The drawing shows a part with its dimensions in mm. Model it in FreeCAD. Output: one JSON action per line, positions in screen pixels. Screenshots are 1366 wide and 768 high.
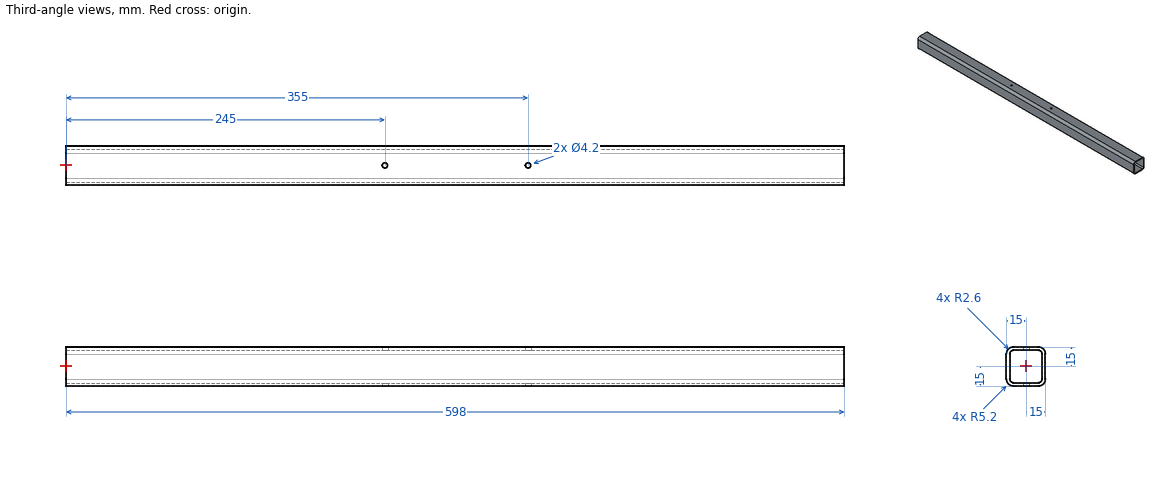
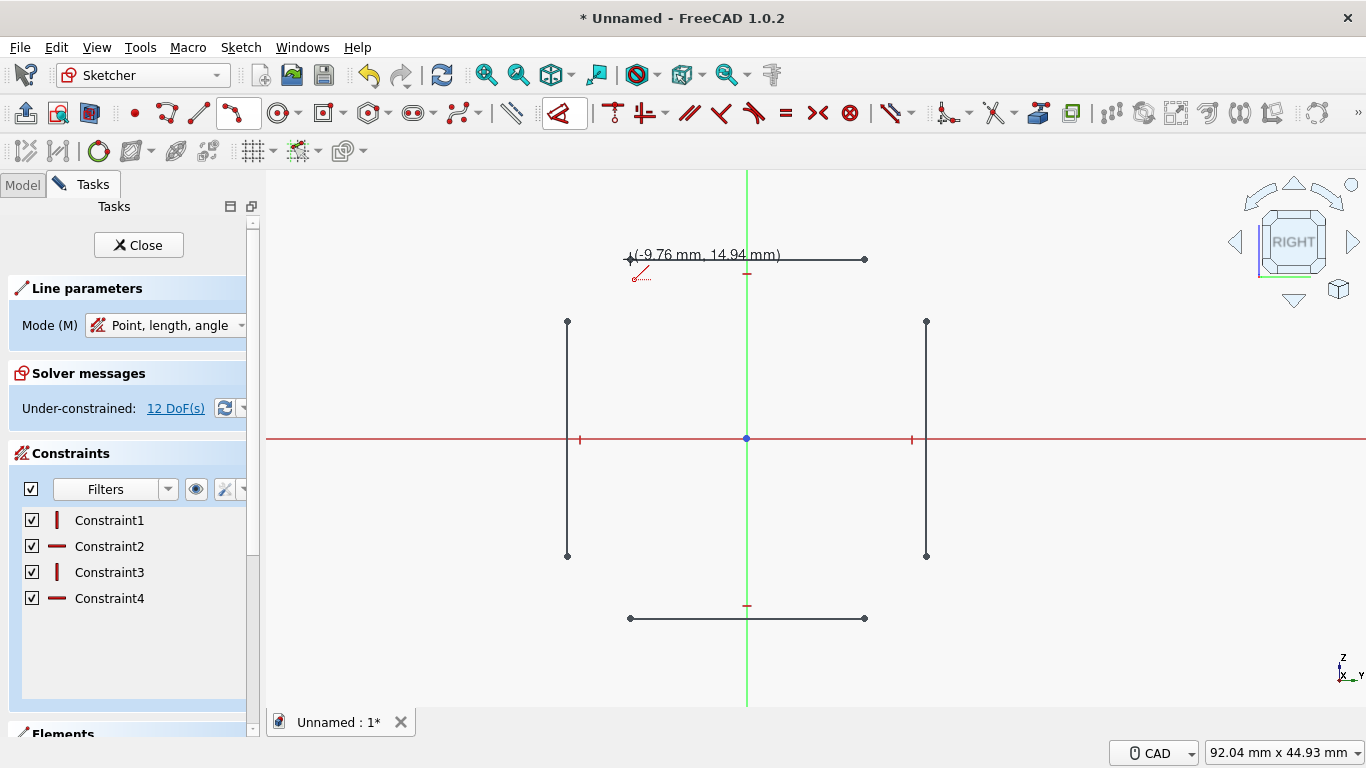
{"action": "left_click", "coordinate": [232, 114]}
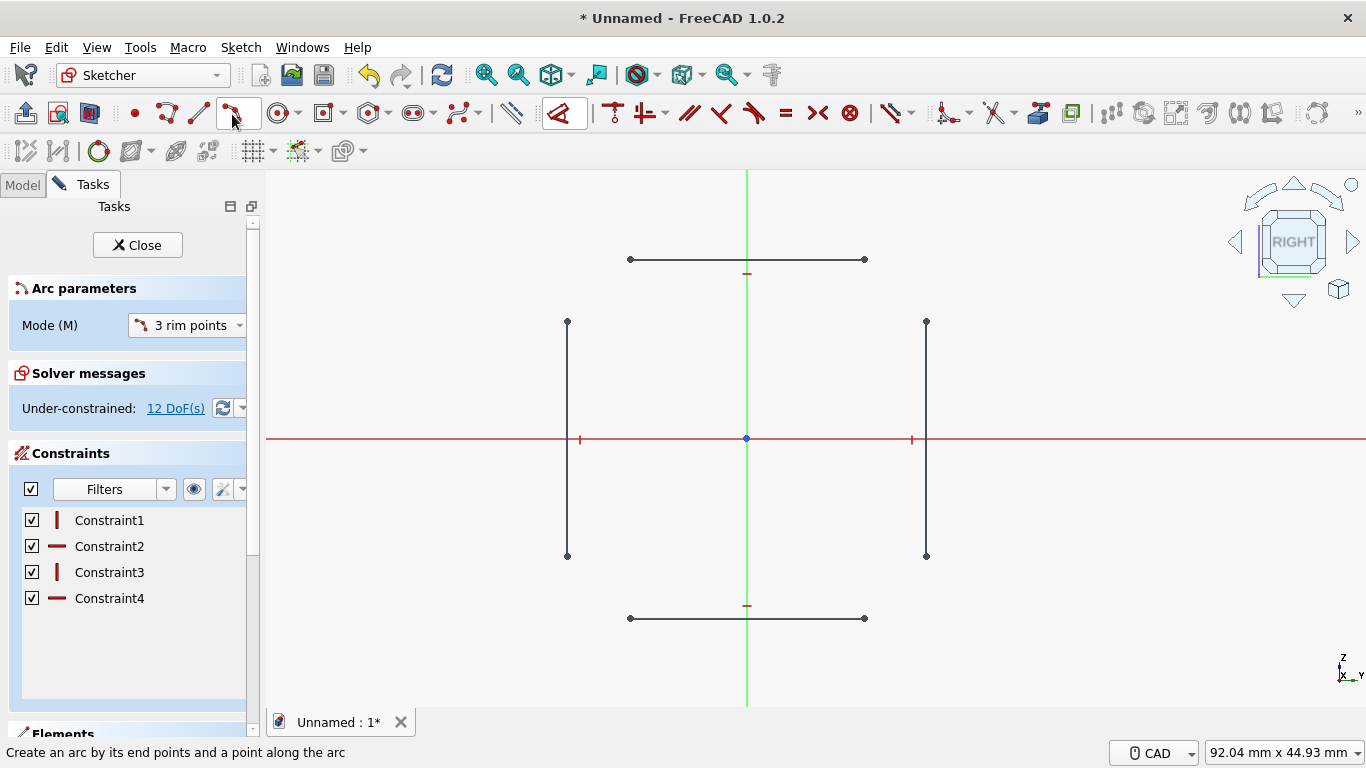
{"action": "left_click", "coordinate": [567, 557]}
{"action": "left_click", "coordinate": [630, 619]}
{"action": "left_click", "coordinate": [586, 600]}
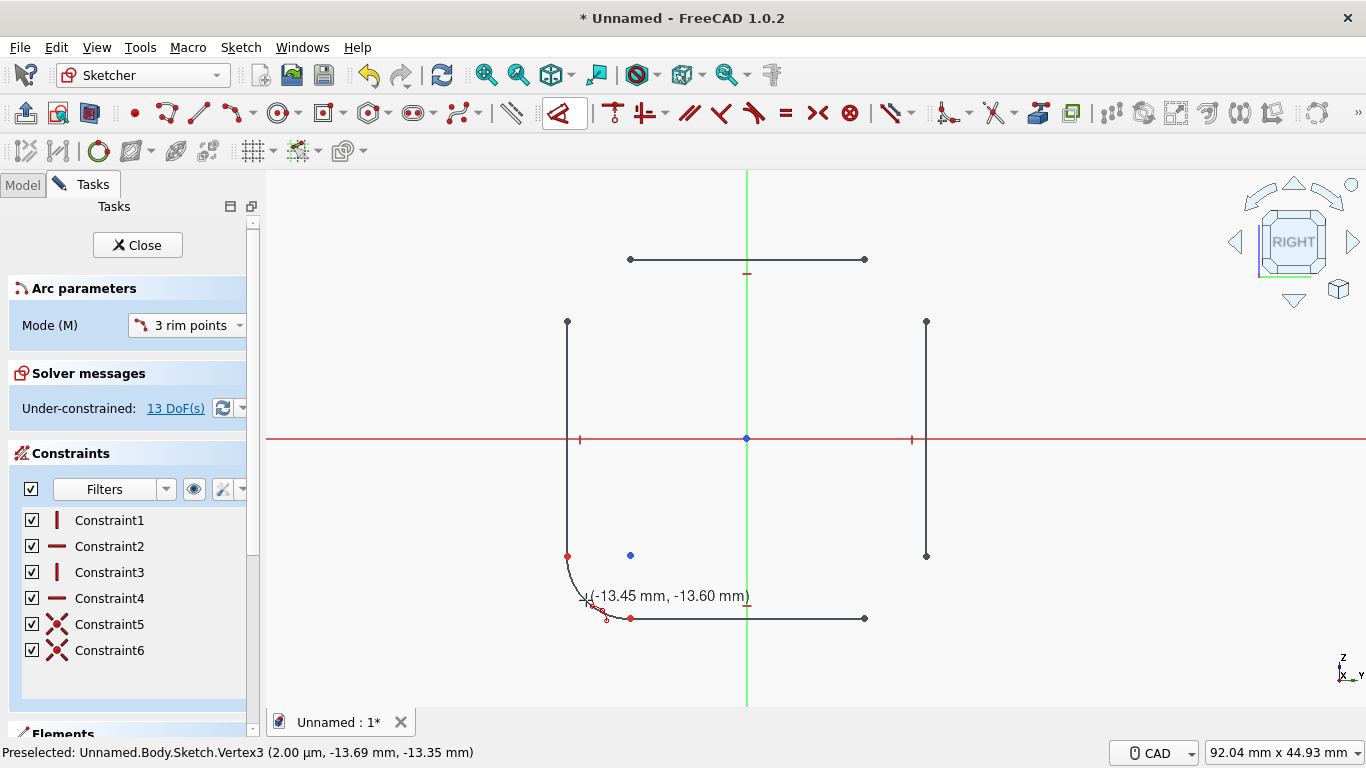
{"action": "left_click", "coordinate": [864, 619]}
{"action": "left_click", "coordinate": [926, 557]}
{"action": "left_click", "coordinate": [908, 600]}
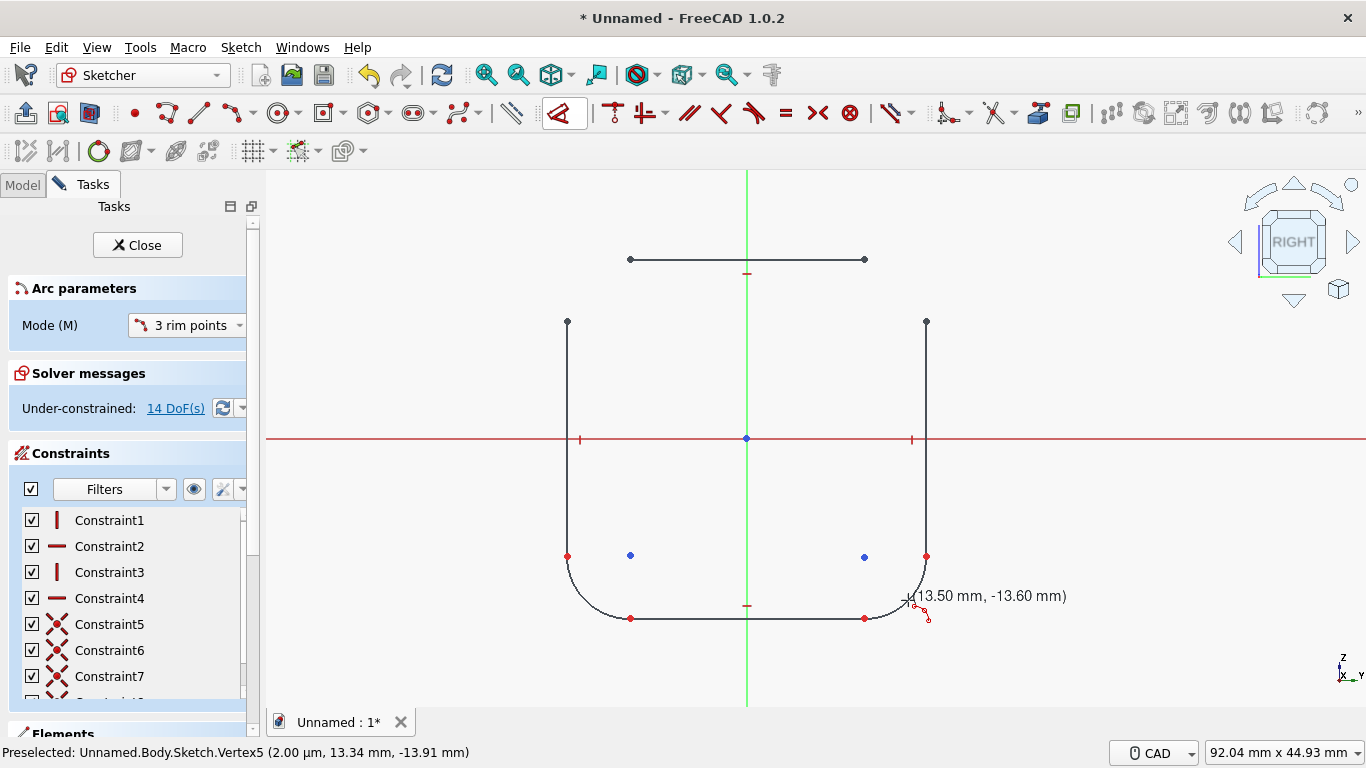
{"action": "left_click", "coordinate": [926, 322]}
{"action": "left_click", "coordinate": [864, 260]}
{"action": "left_click", "coordinate": [908, 277]}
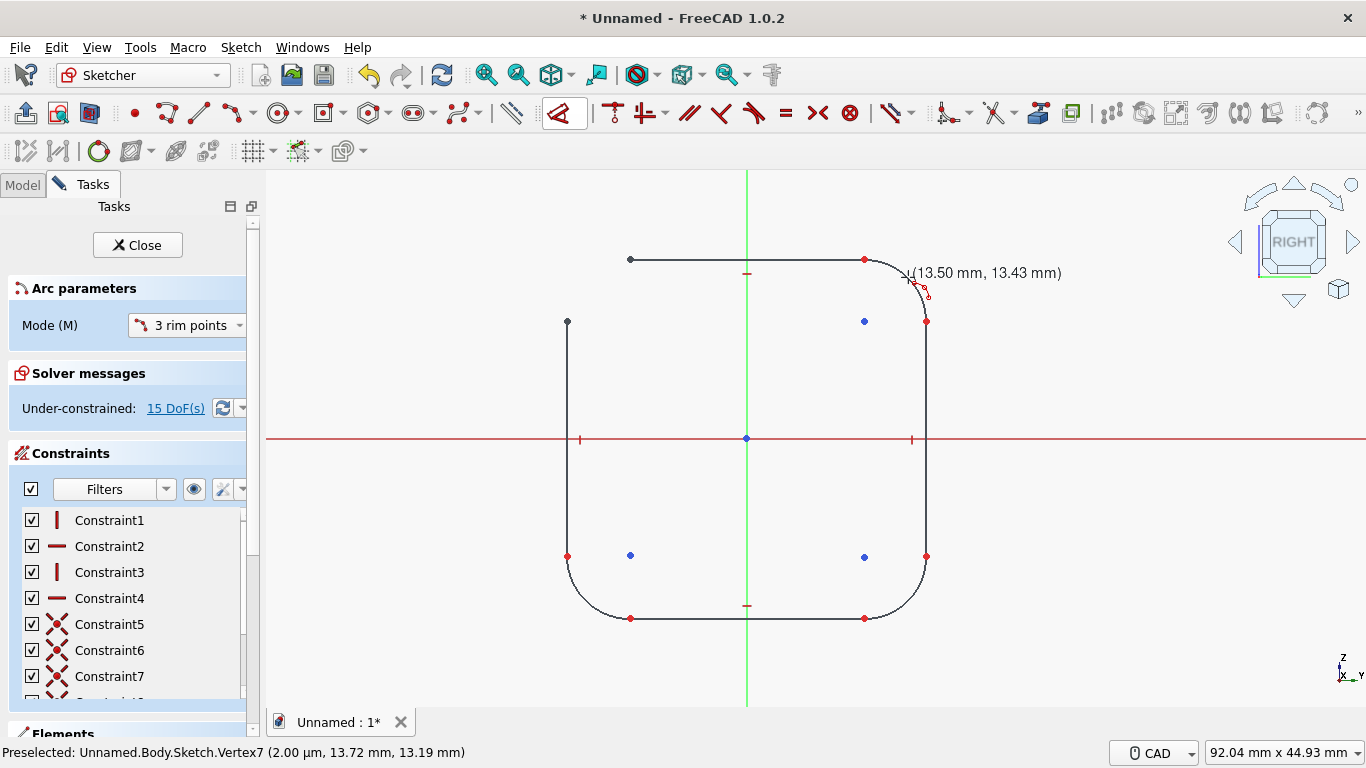
{"action": "left_click", "coordinate": [630, 260]}
{"action": "left_click", "coordinate": [567, 322]}
{"action": "left_click", "coordinate": [586, 277]}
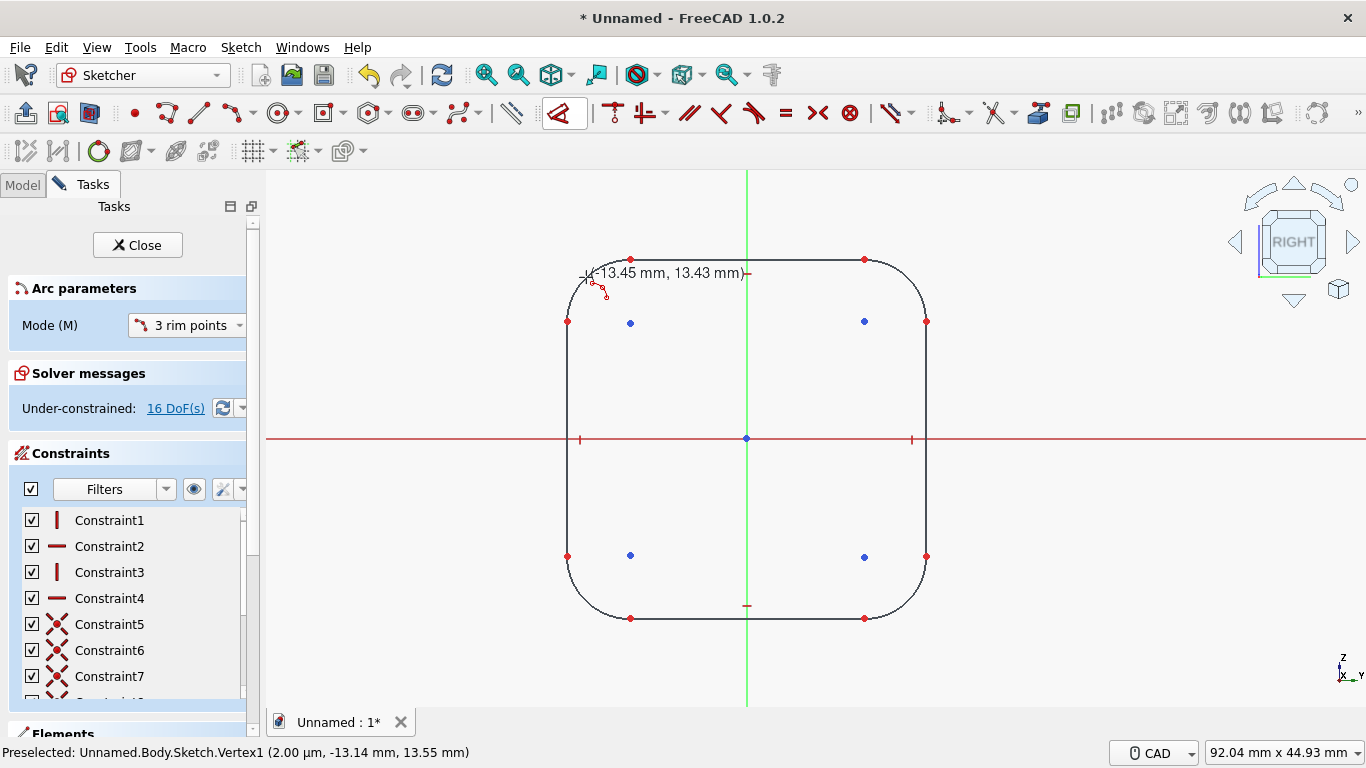
{"action": "key", "text": "g l"}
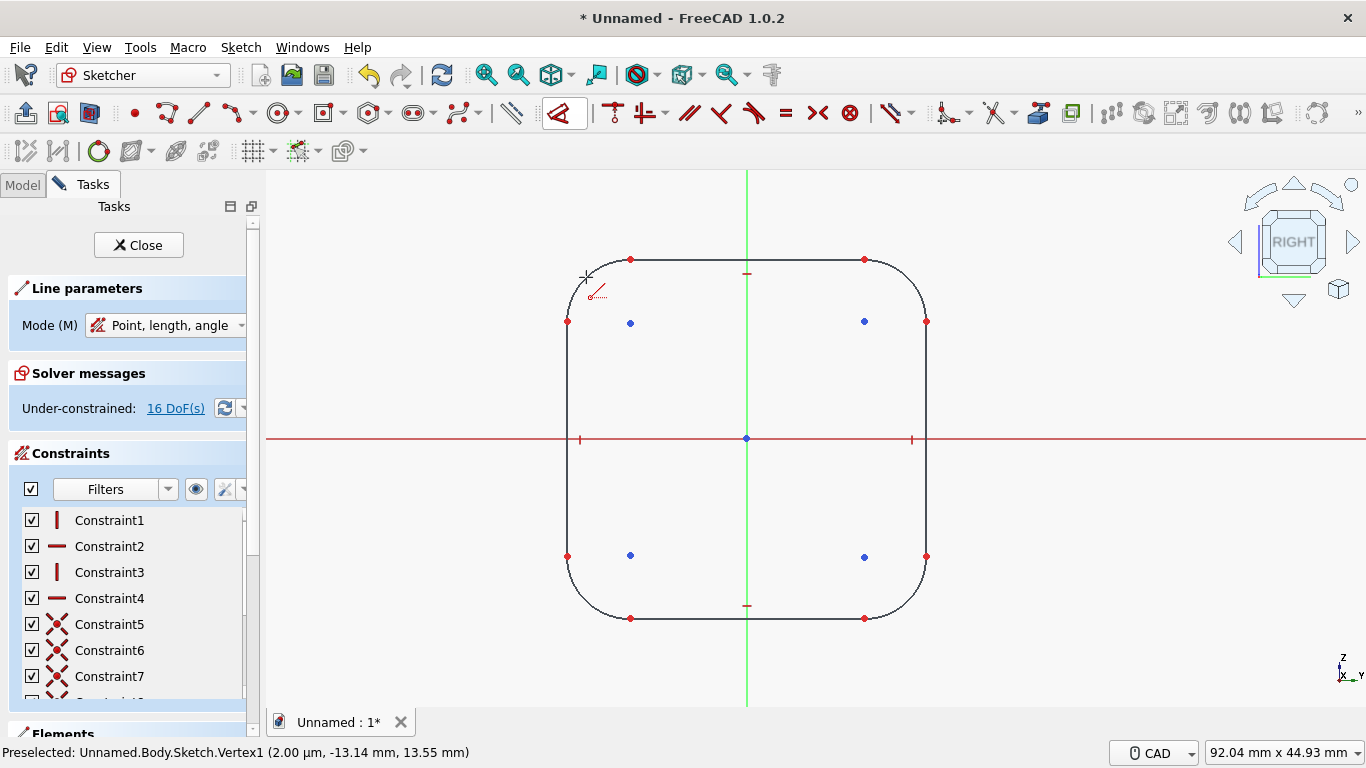
{"action": "left_click", "coordinate": [598, 556]}
{"action": "left_click", "coordinate": [598, 321]}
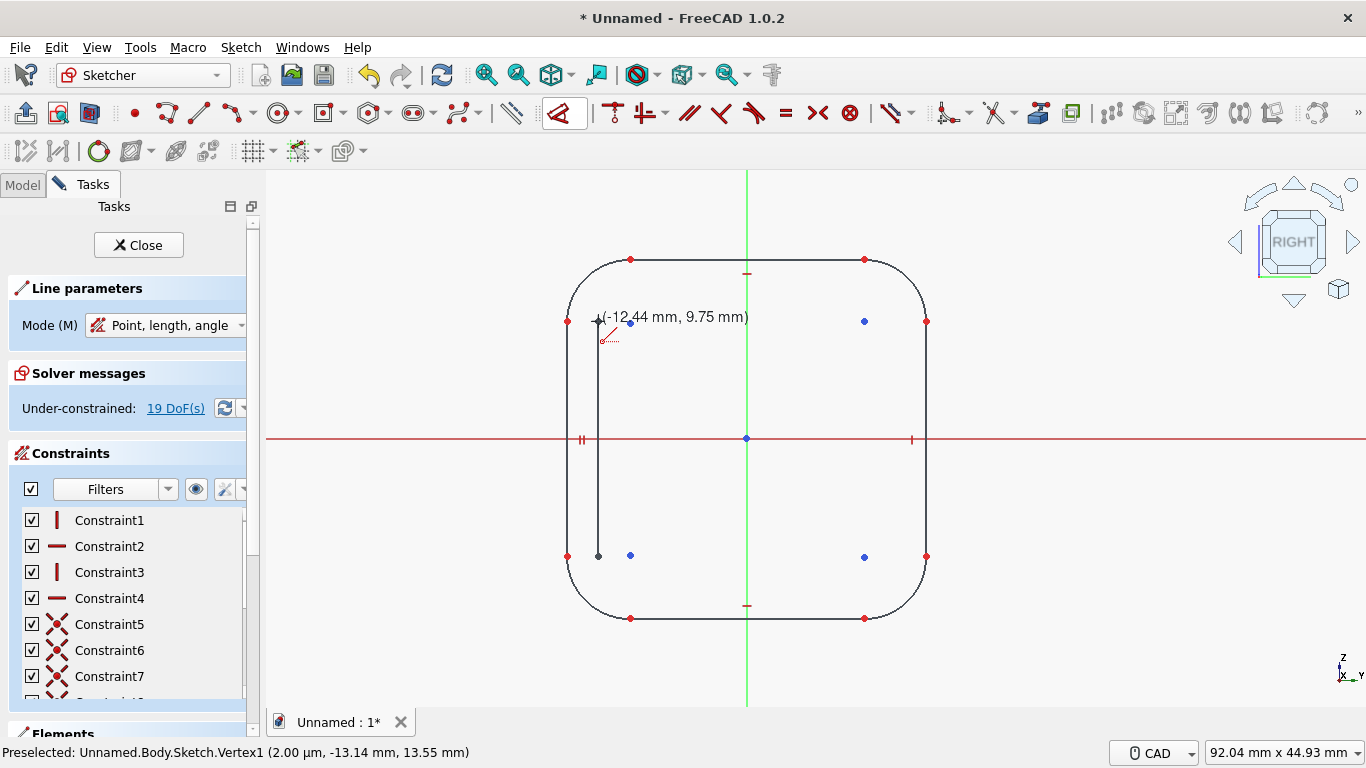
{"action": "left_click", "coordinate": [630, 290]}
{"action": "left_click", "coordinate": [864, 290]}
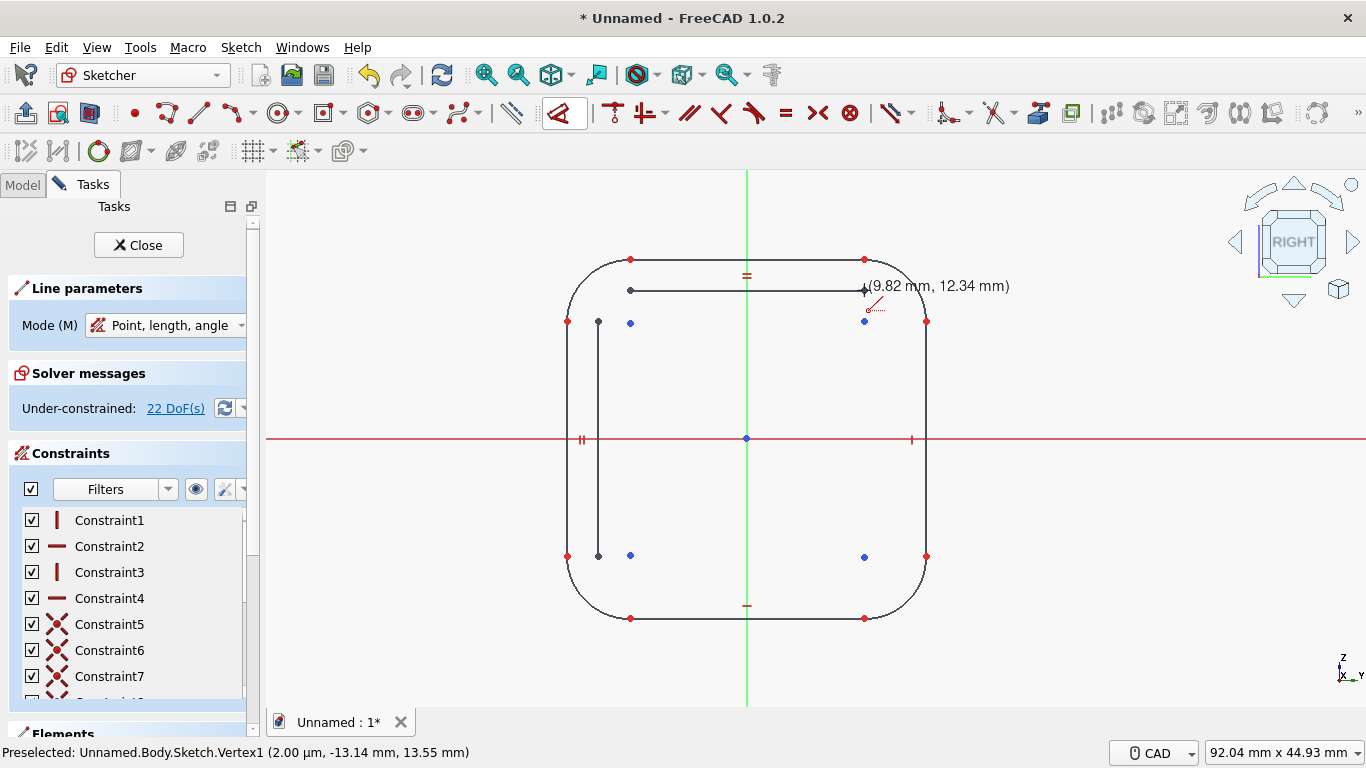
{"action": "left_click", "coordinate": [895, 321]}
{"action": "left_click", "coordinate": [895, 556]}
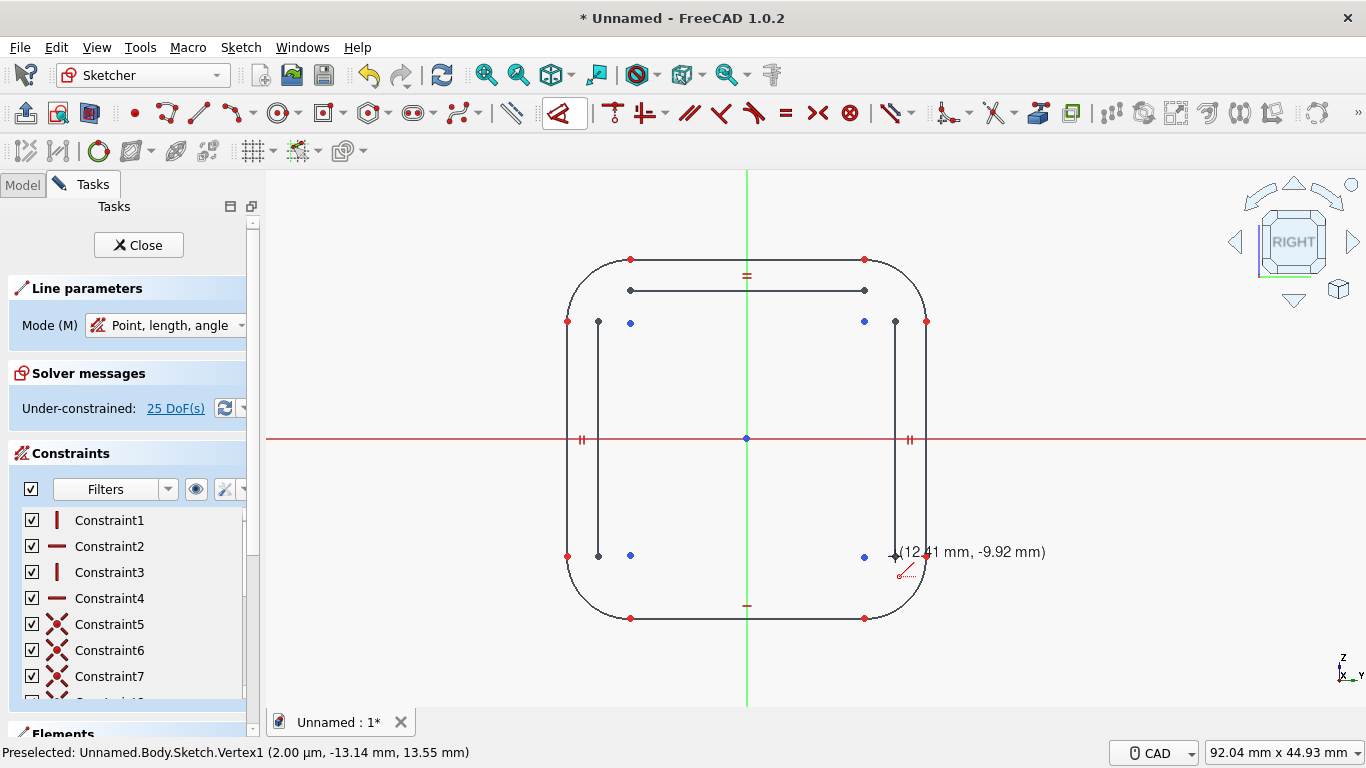
{"action": "left_click", "coordinate": [864, 587]}
{"action": "left_click", "coordinate": [630, 587]}